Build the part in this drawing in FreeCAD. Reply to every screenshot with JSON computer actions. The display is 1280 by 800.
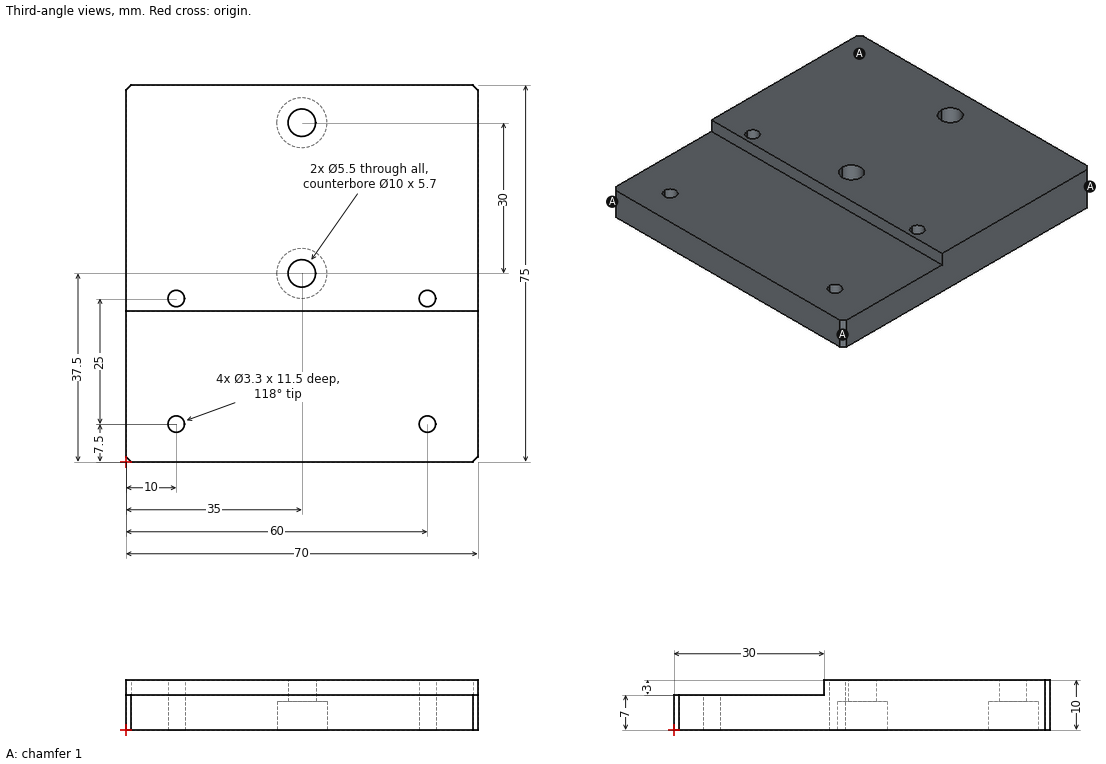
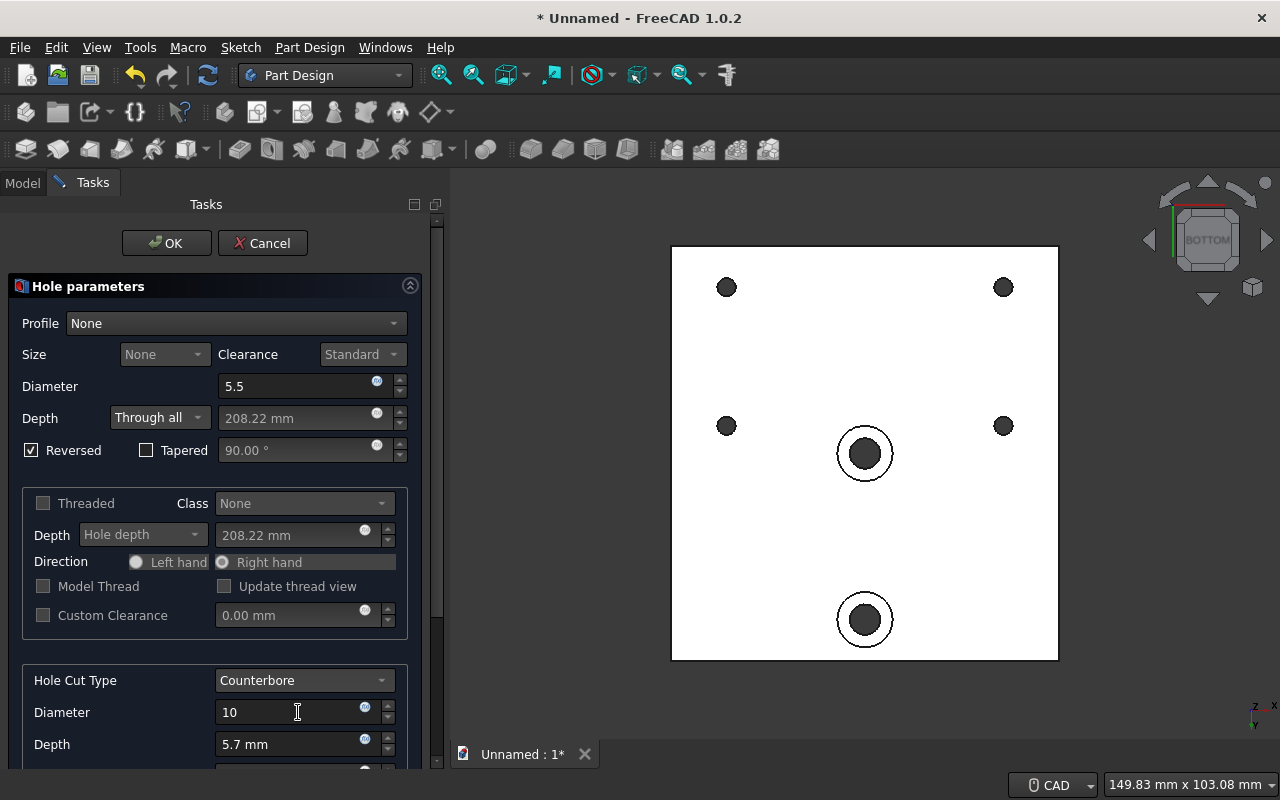
{"action": "left_click", "coordinate": [167, 243]}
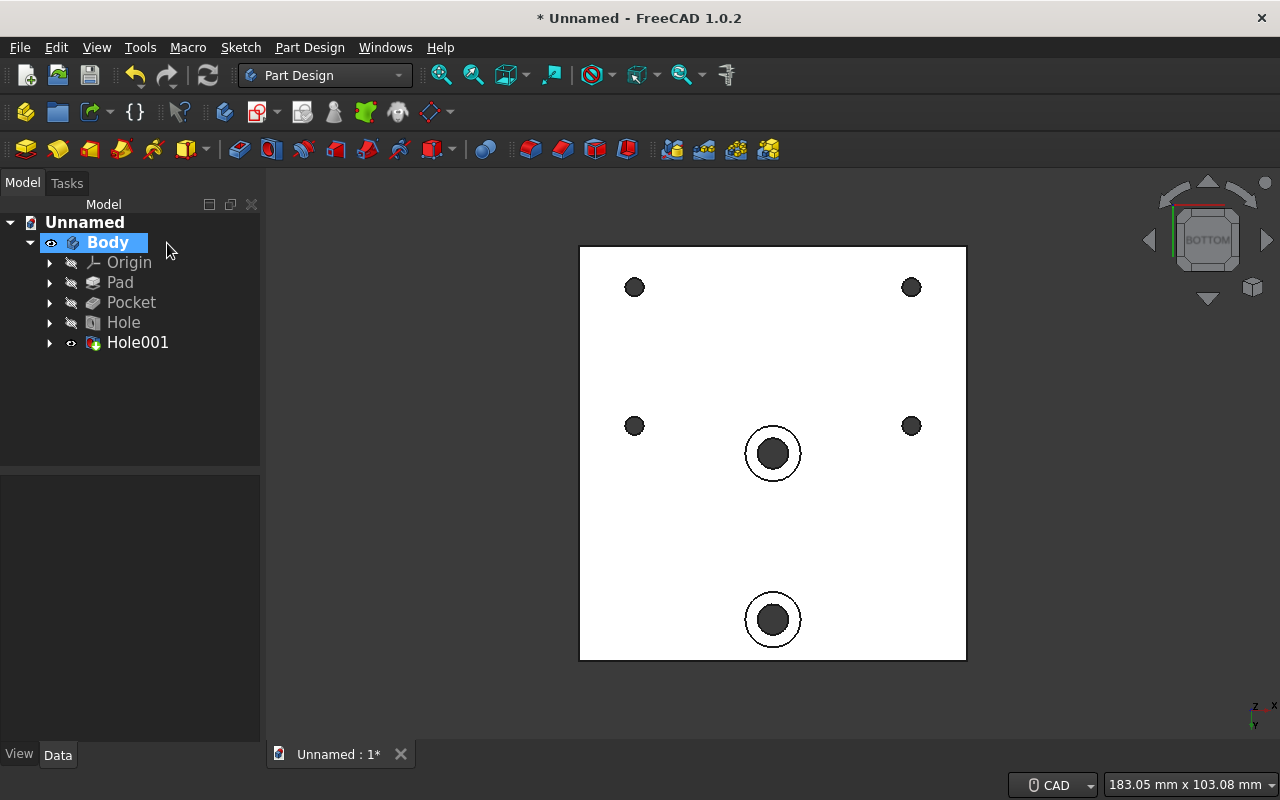
{"action": "key", "text": "0"}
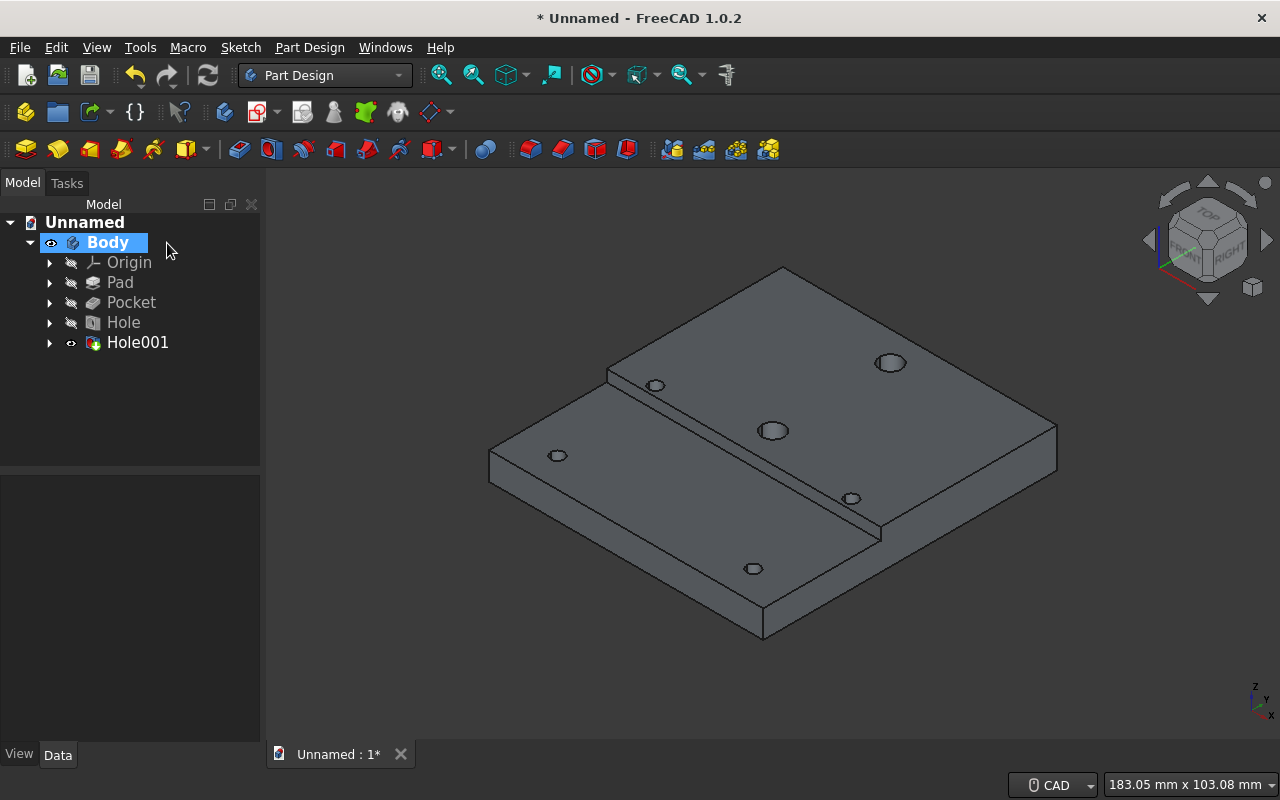
{"action": "left_click", "coordinate": [763, 623]}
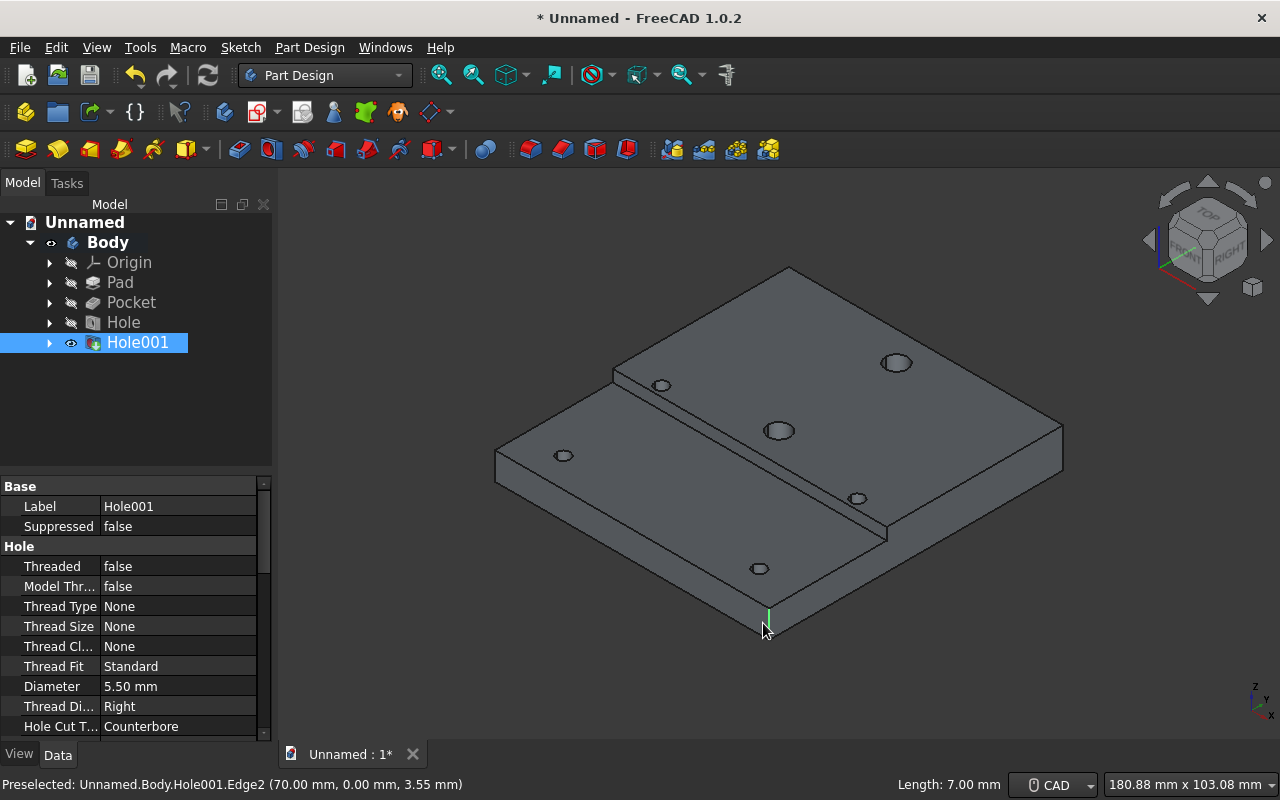
{"action": "key", "text": "2"}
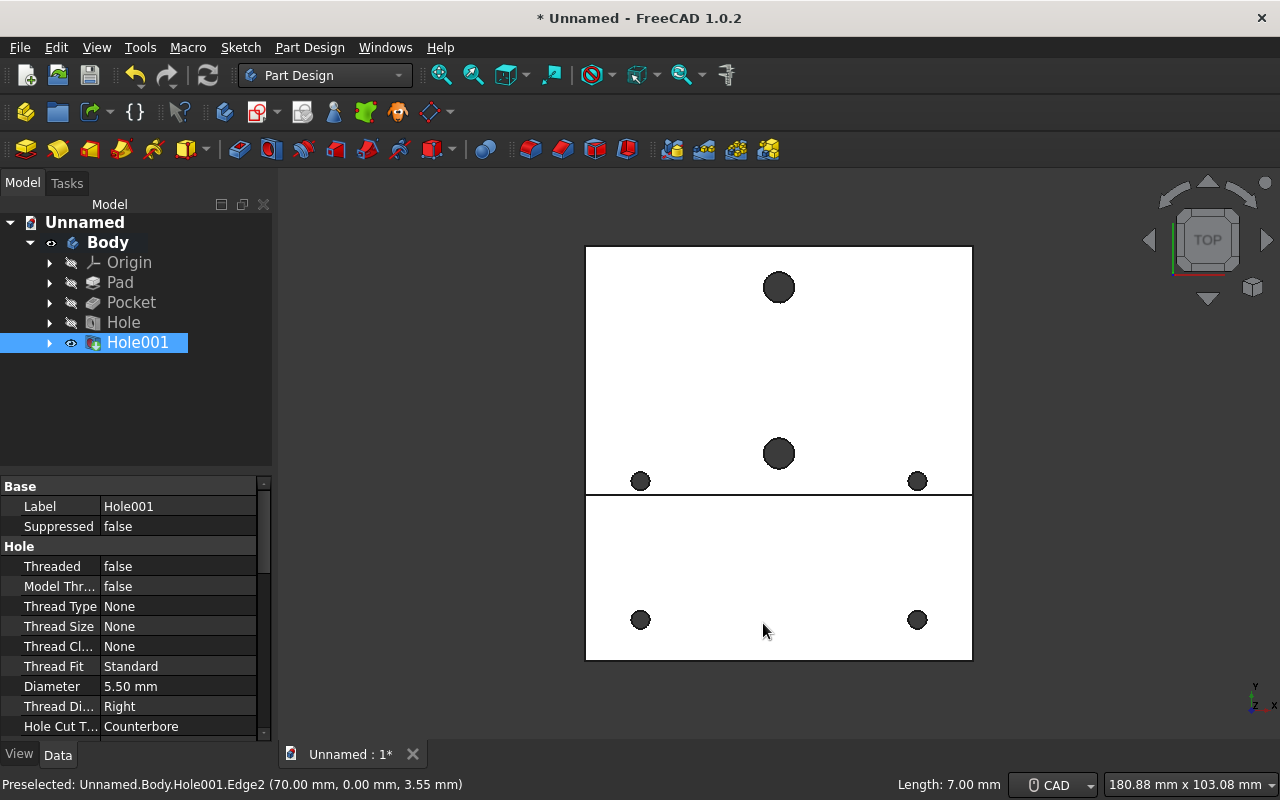
{"action": "key", "text": "1"}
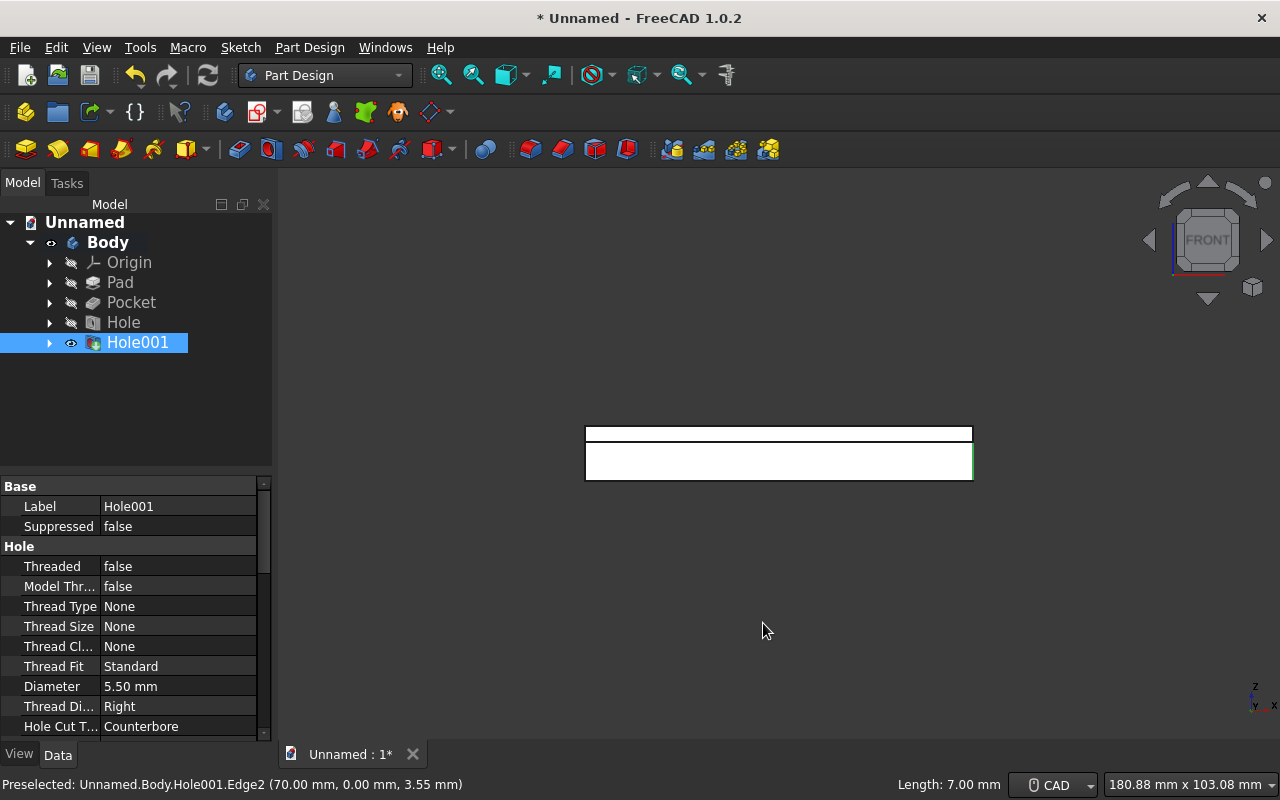
{"action": "left_click", "coordinate": [442, 76]}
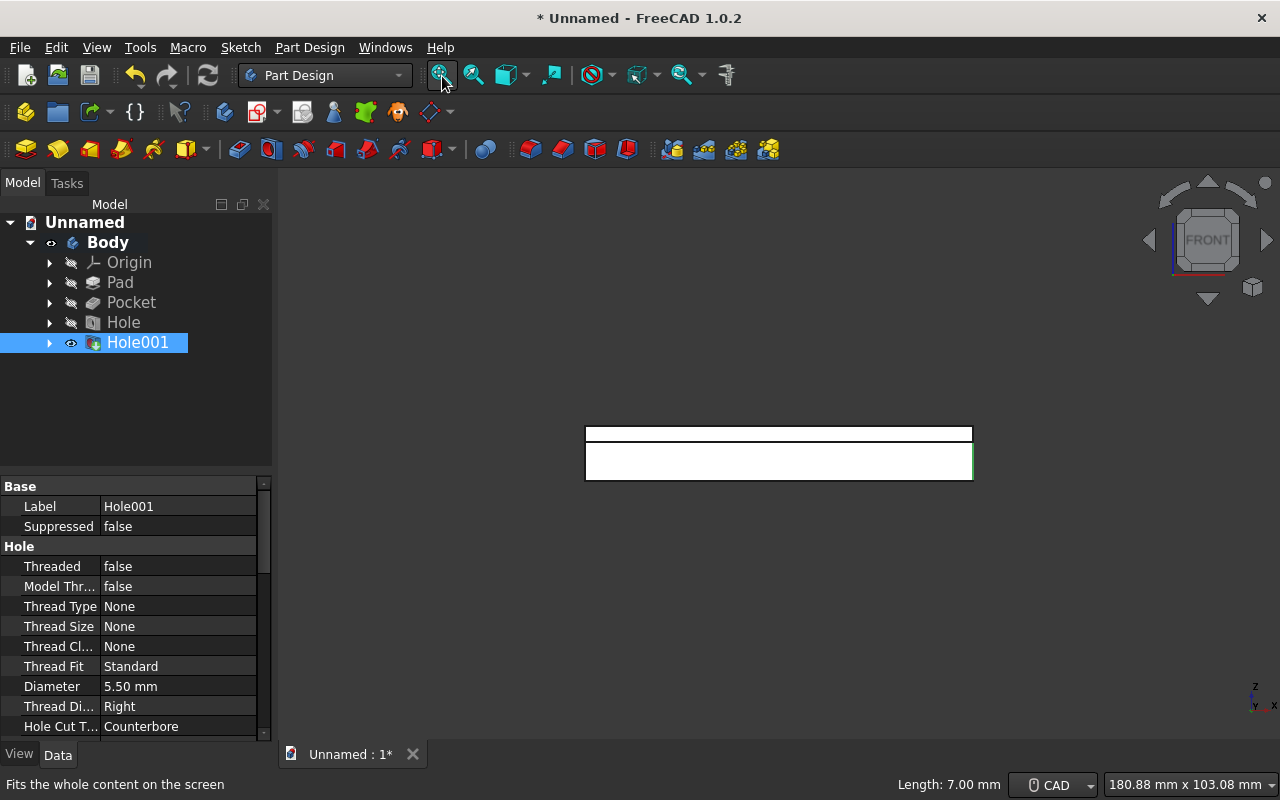
{"action": "left_click", "coordinate": [585, 461], "text": "ctrl"}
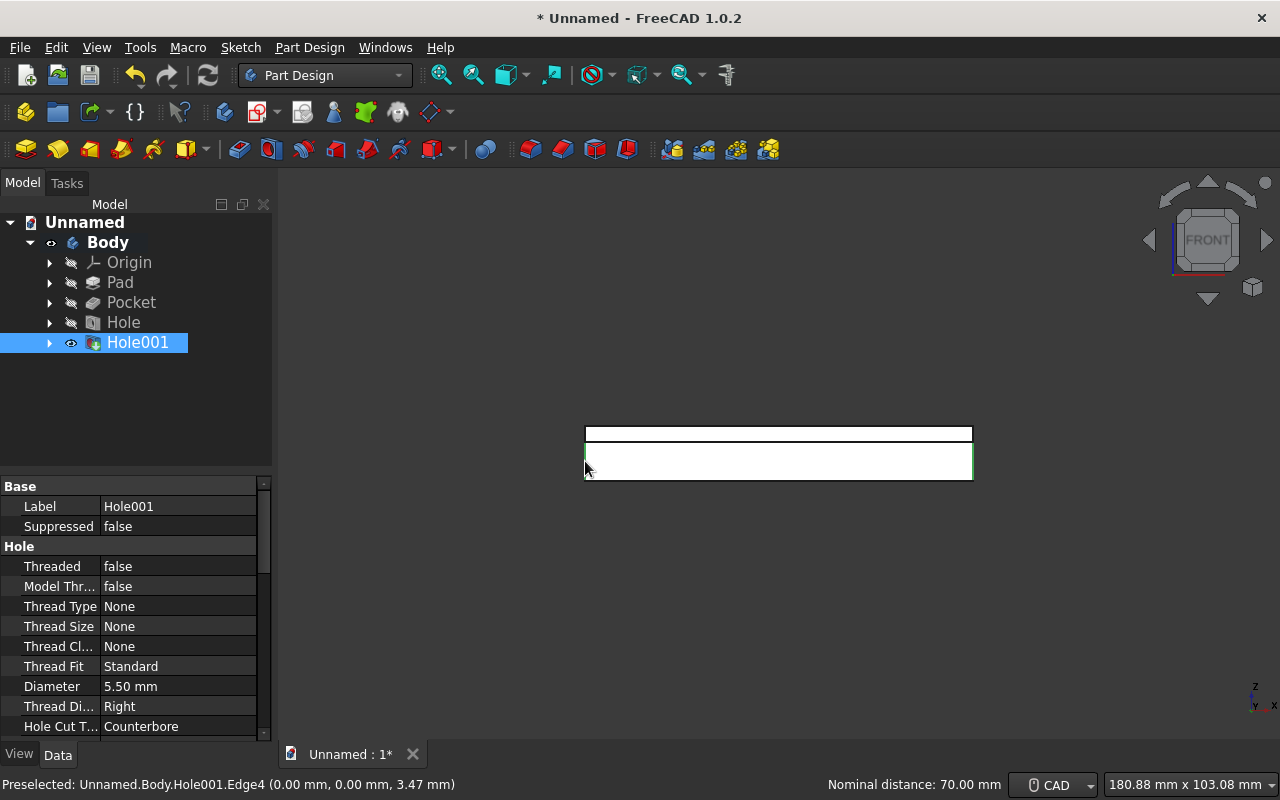
{"action": "key", "text": "3"}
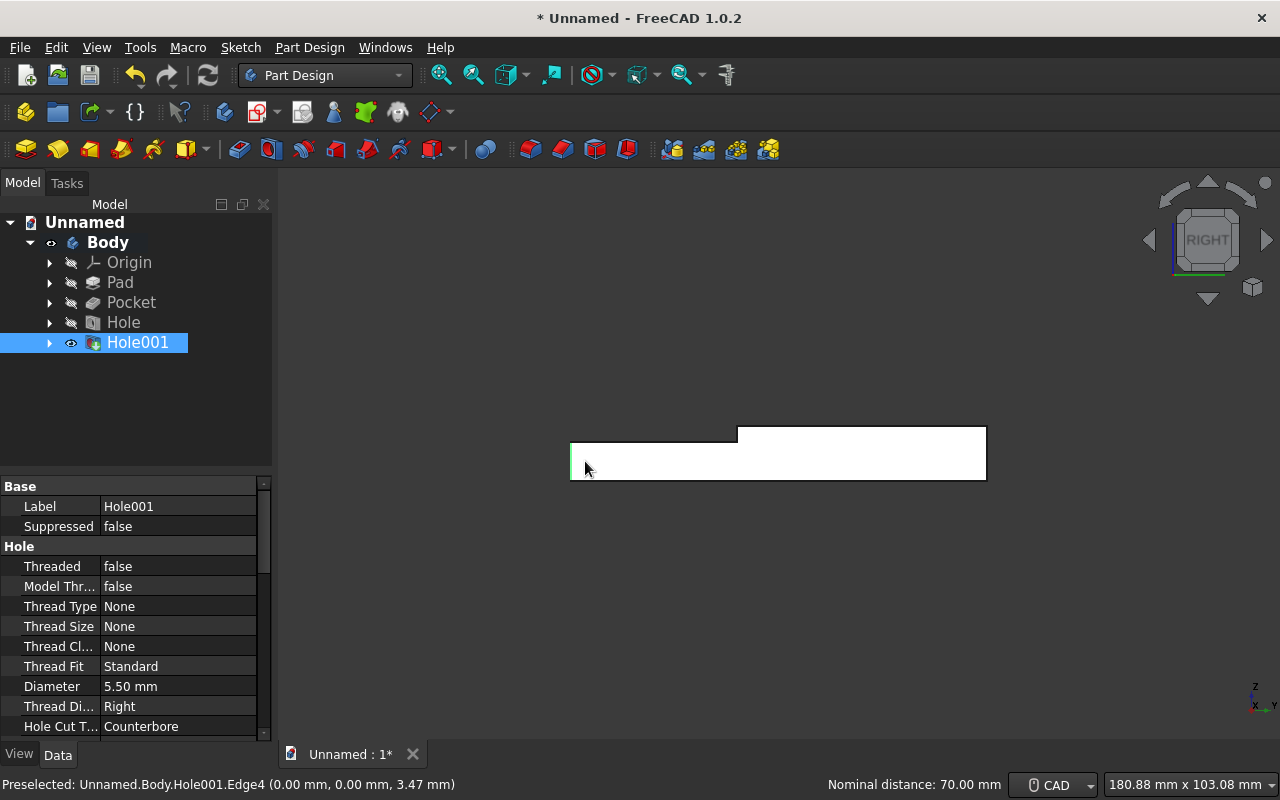
{"action": "left_click", "coordinate": [442, 76]}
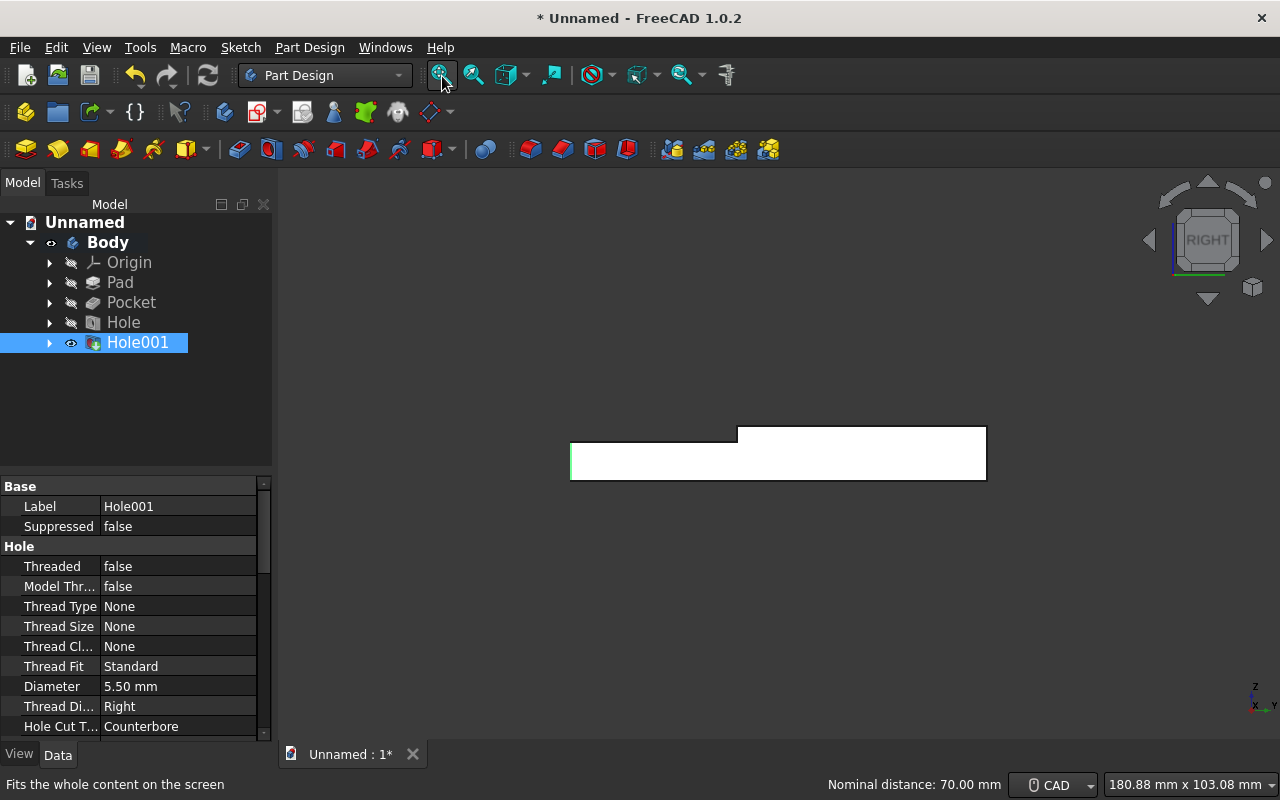
{"action": "left_click", "coordinate": [987, 452], "text": "ctrl"}